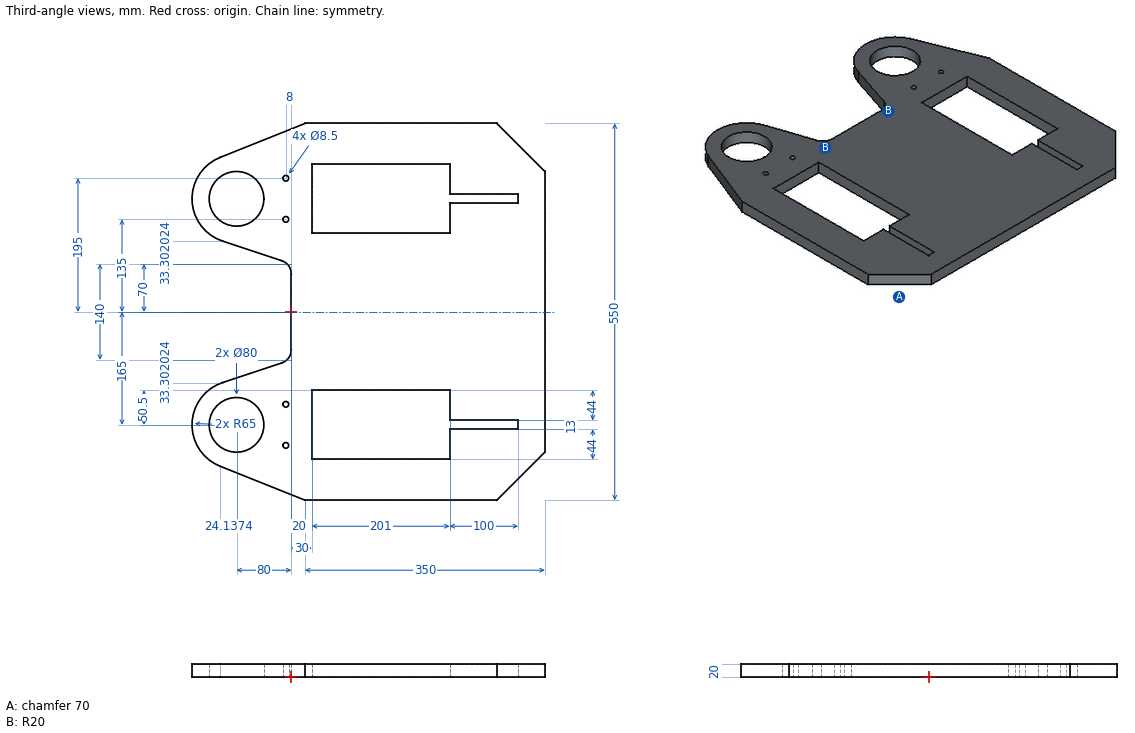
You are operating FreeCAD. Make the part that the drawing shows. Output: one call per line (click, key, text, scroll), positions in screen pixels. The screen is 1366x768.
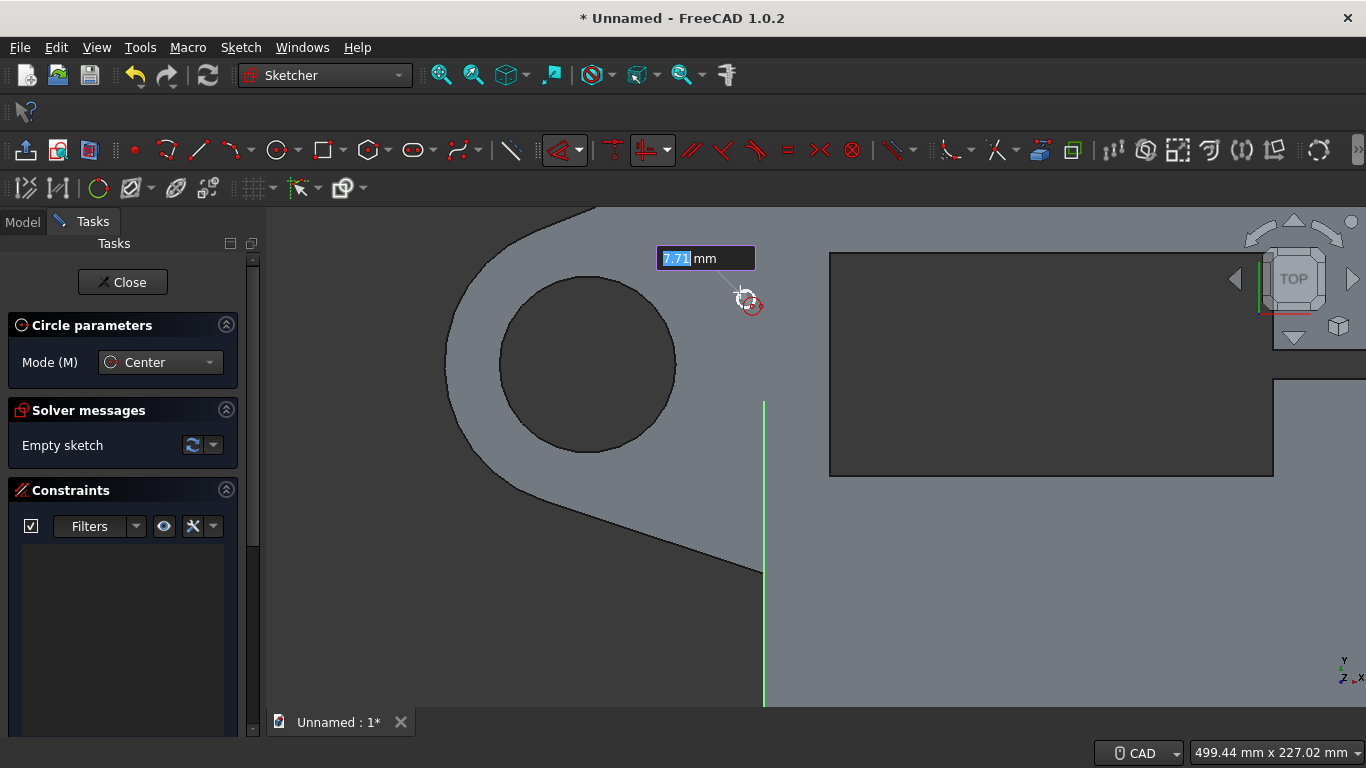
text(8.5)
key(Return)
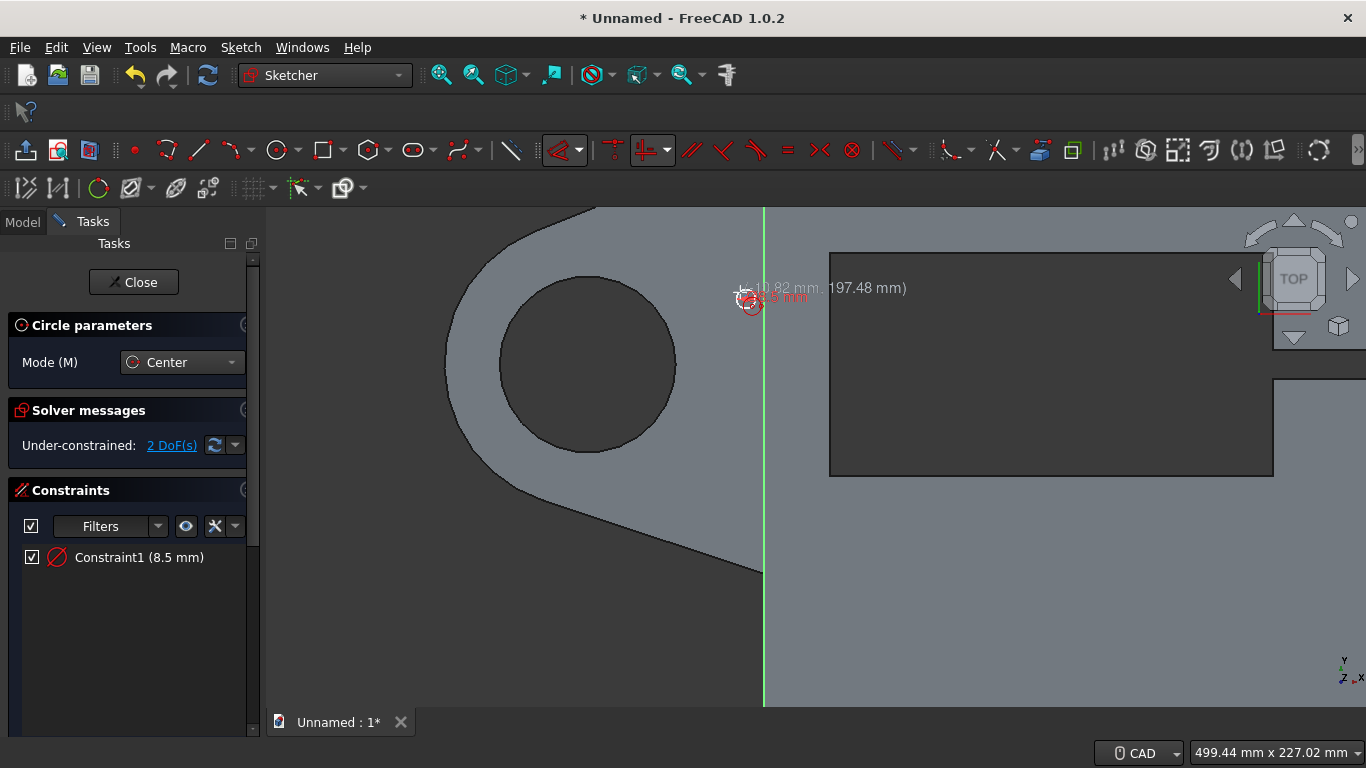
scroll(746, 431, up, 5)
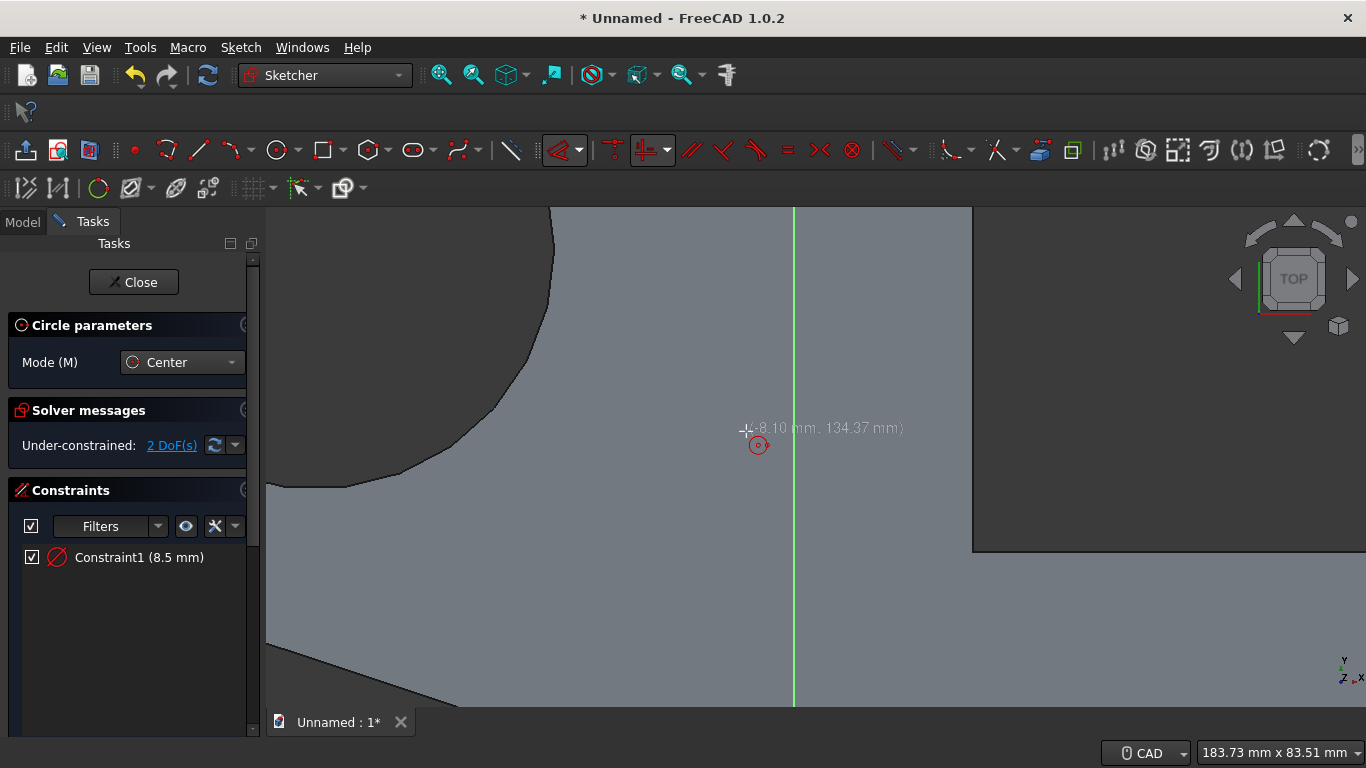
scroll(746, 335, down, 10)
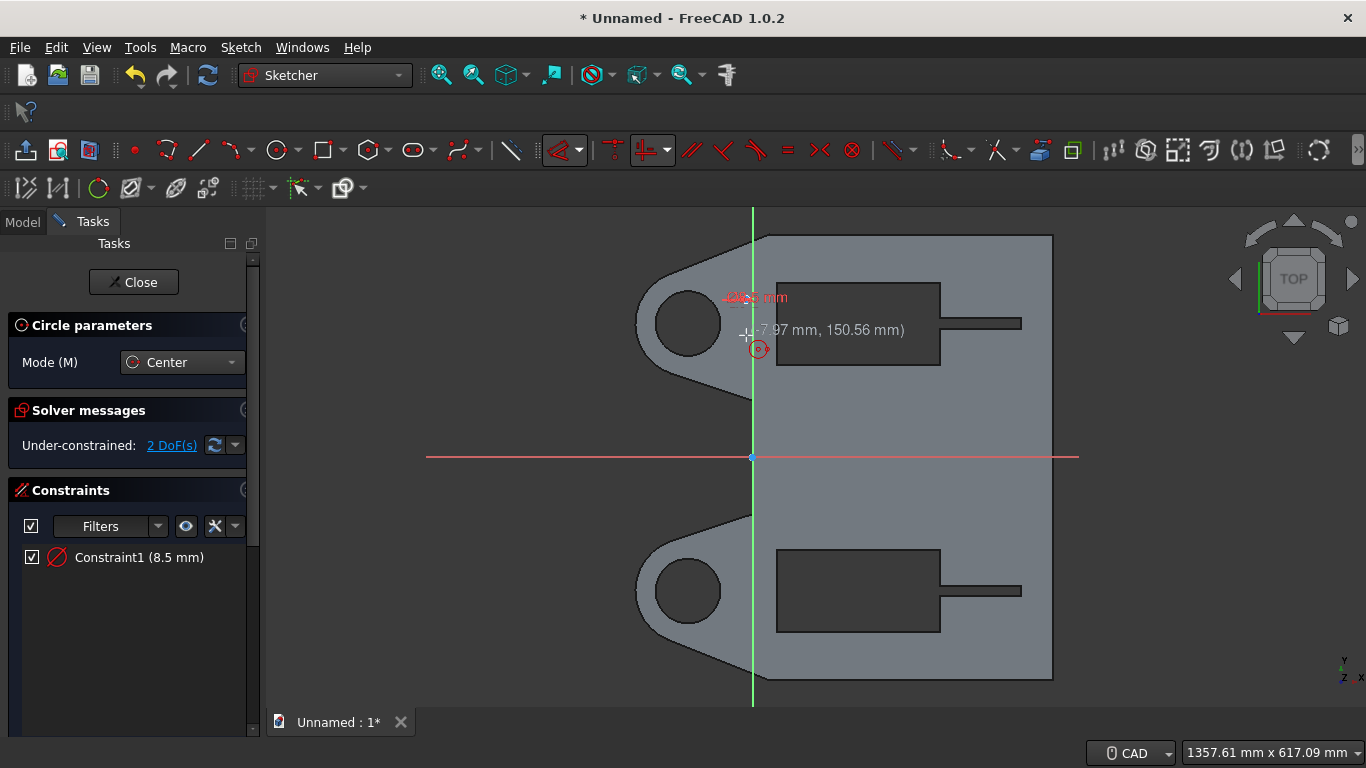
scroll(746, 348, up, 5)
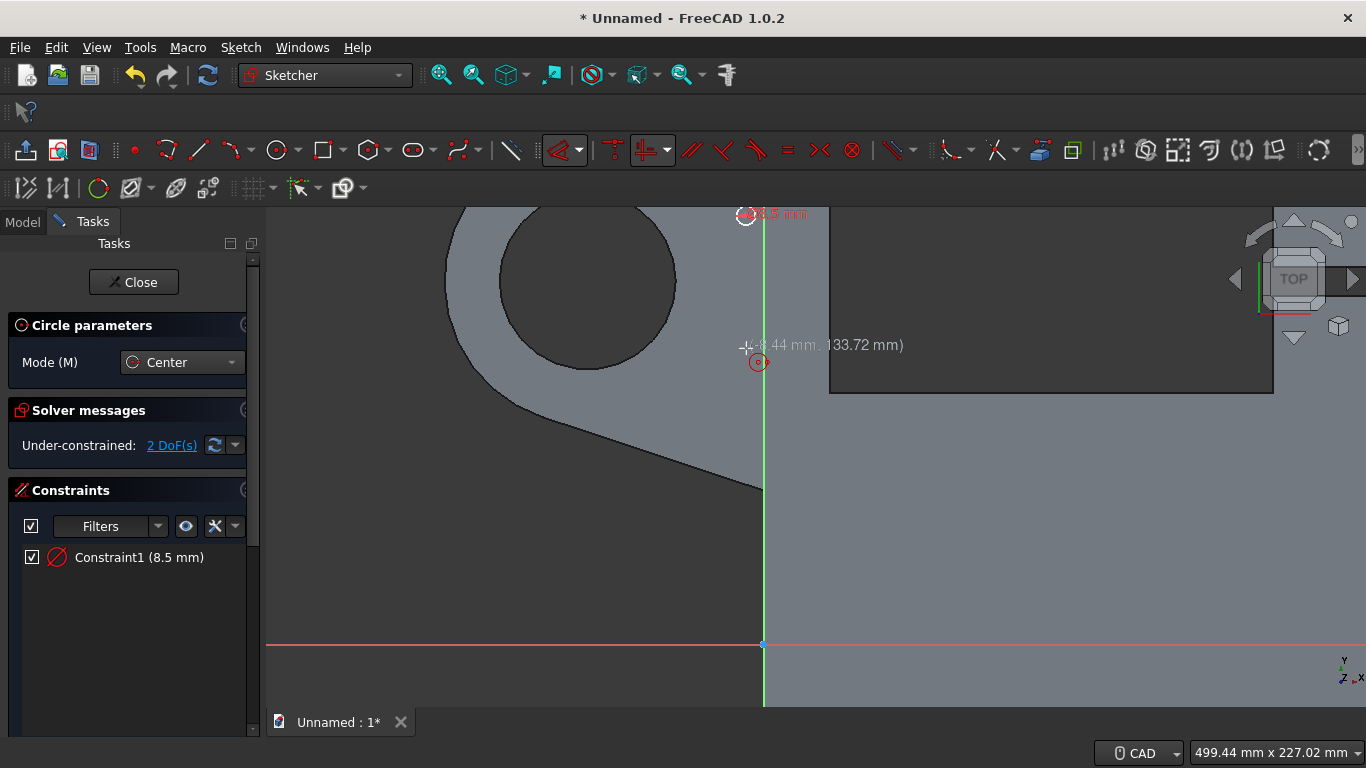
click(746, 347)
move(740, 341)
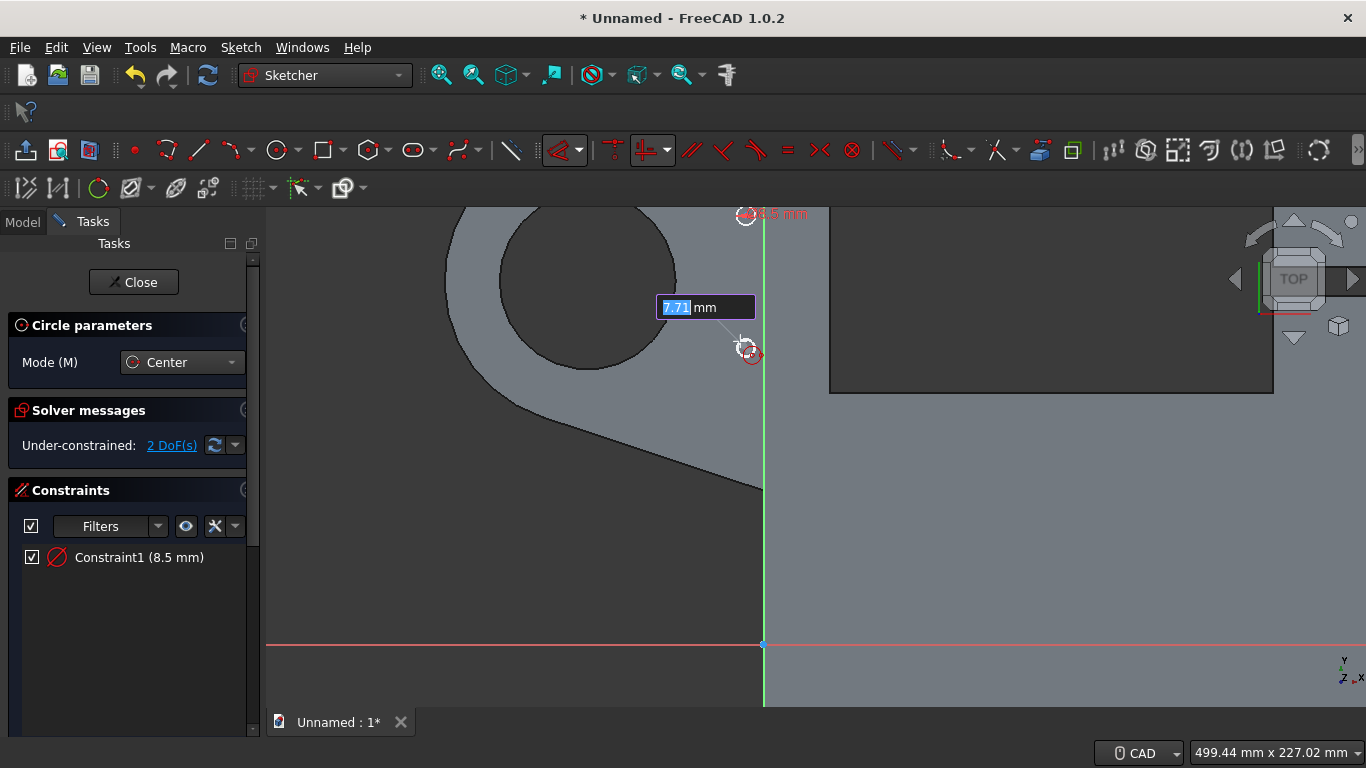
text(8.5)
key(Return)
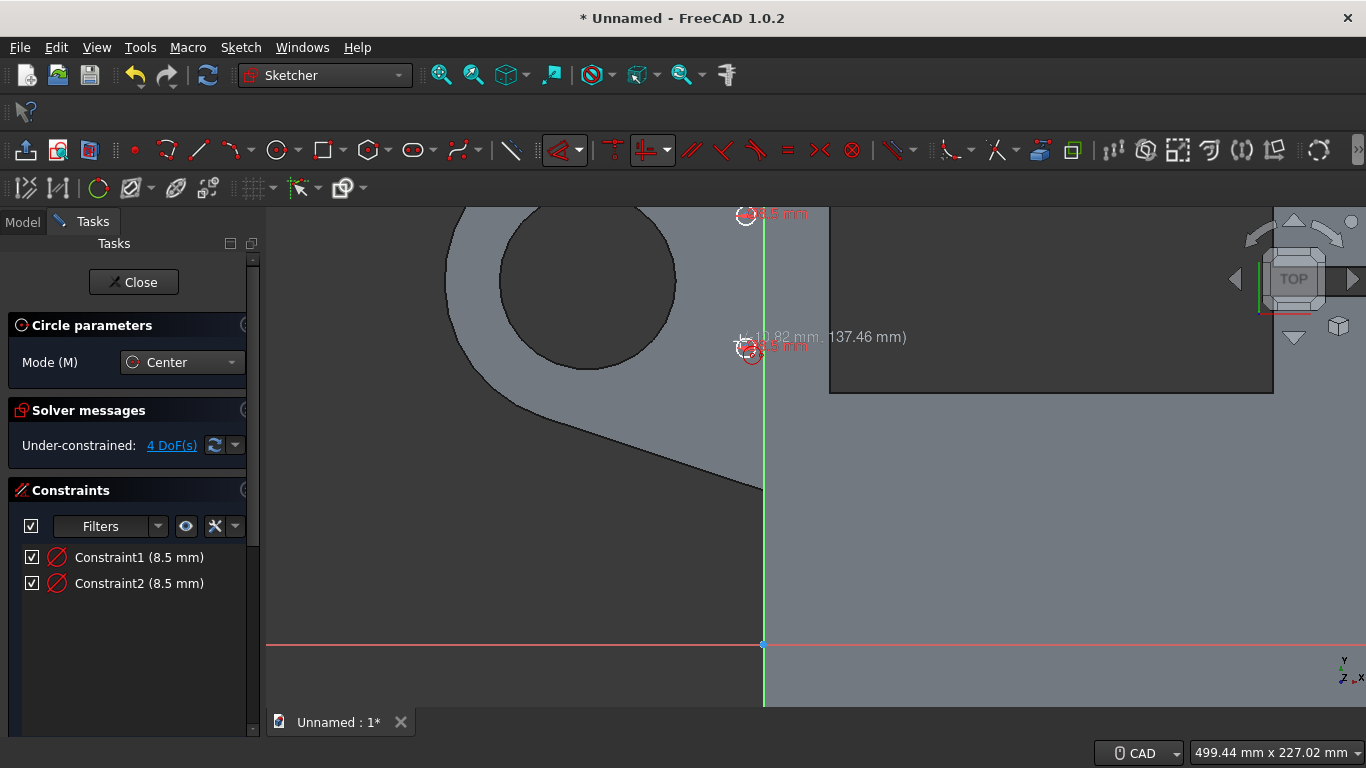
scroll(746, 348, down, 5)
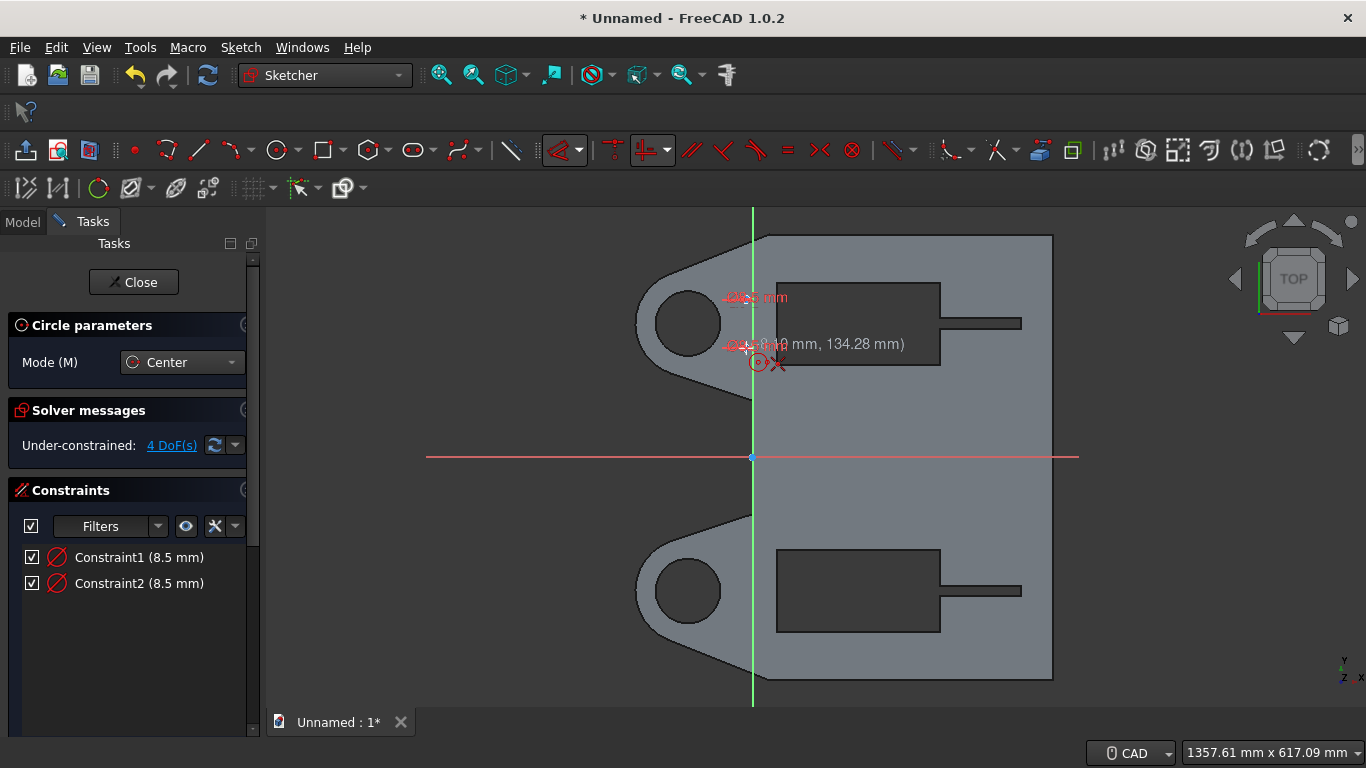
scroll(746, 567, up, 10)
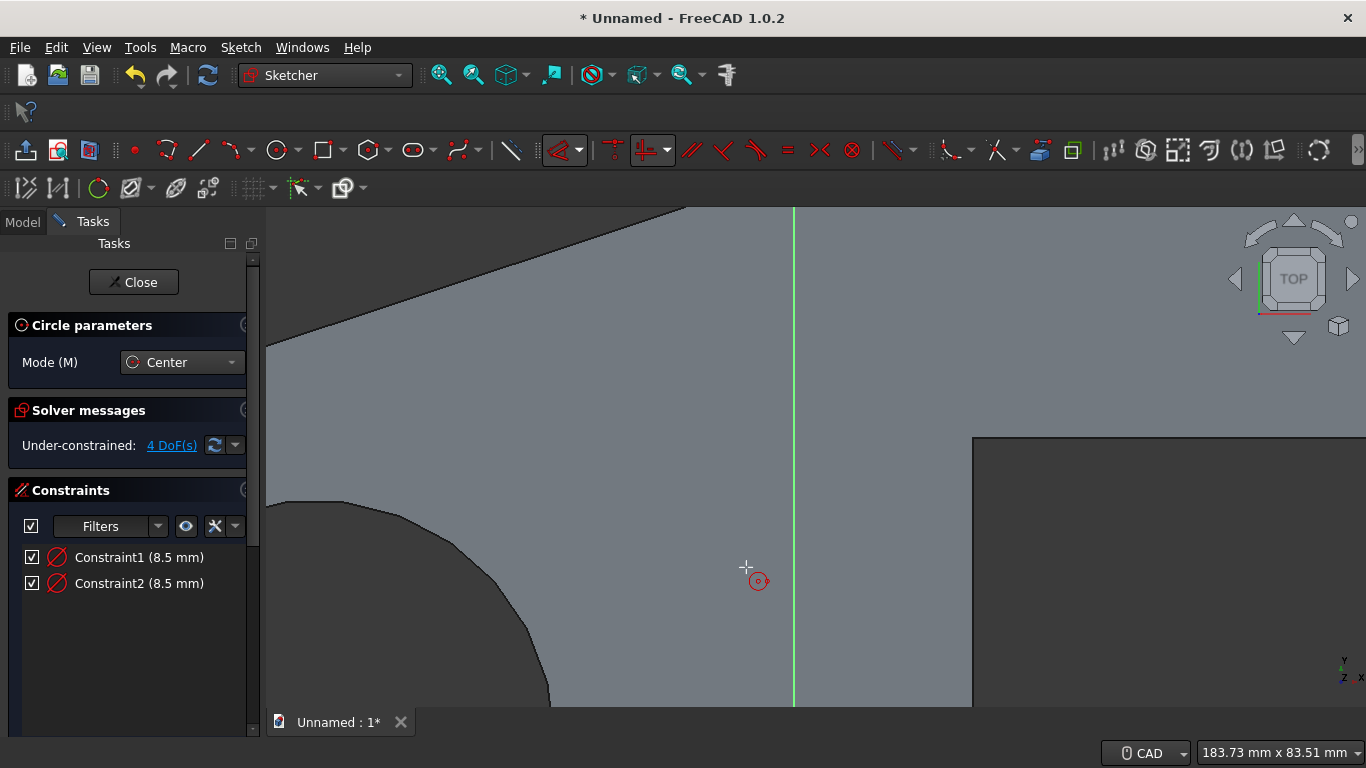
scroll(746, 567, down, 10)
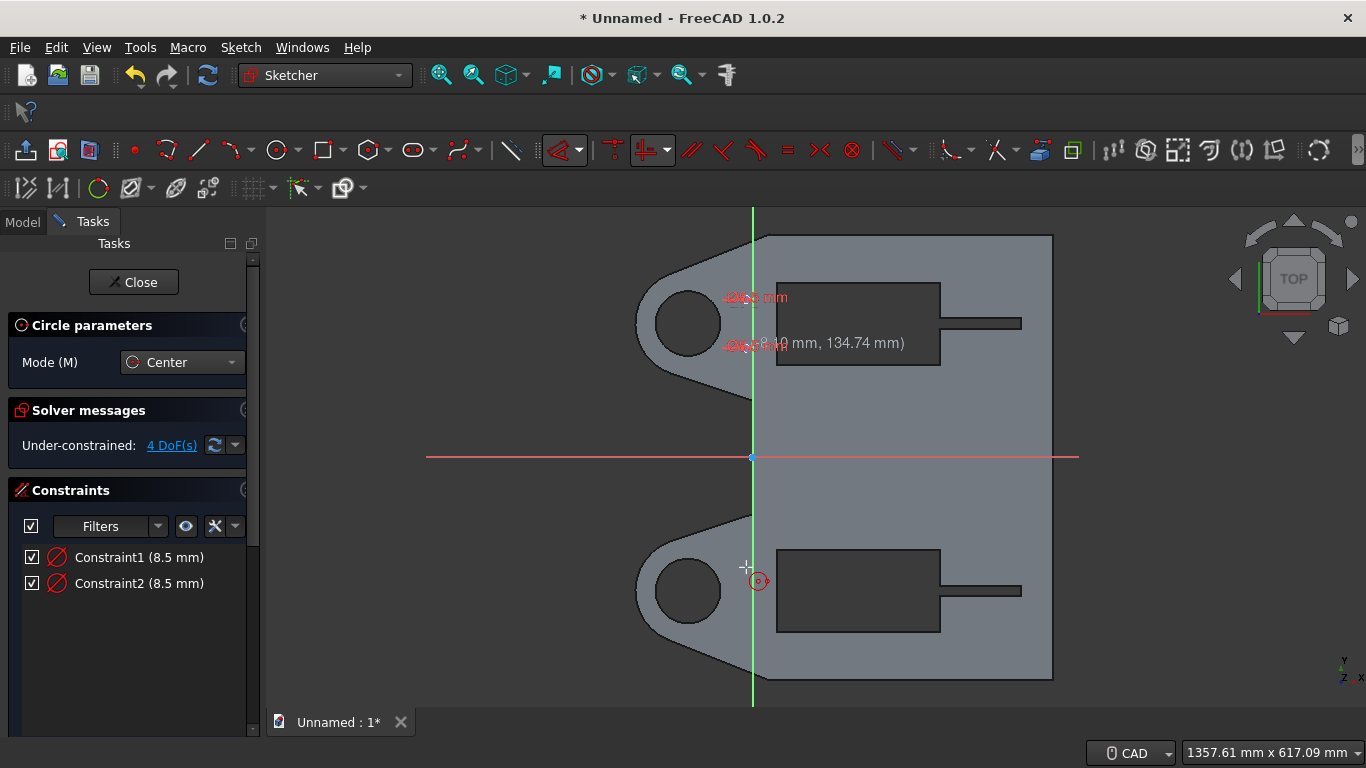
scroll(746, 567, up, 5)